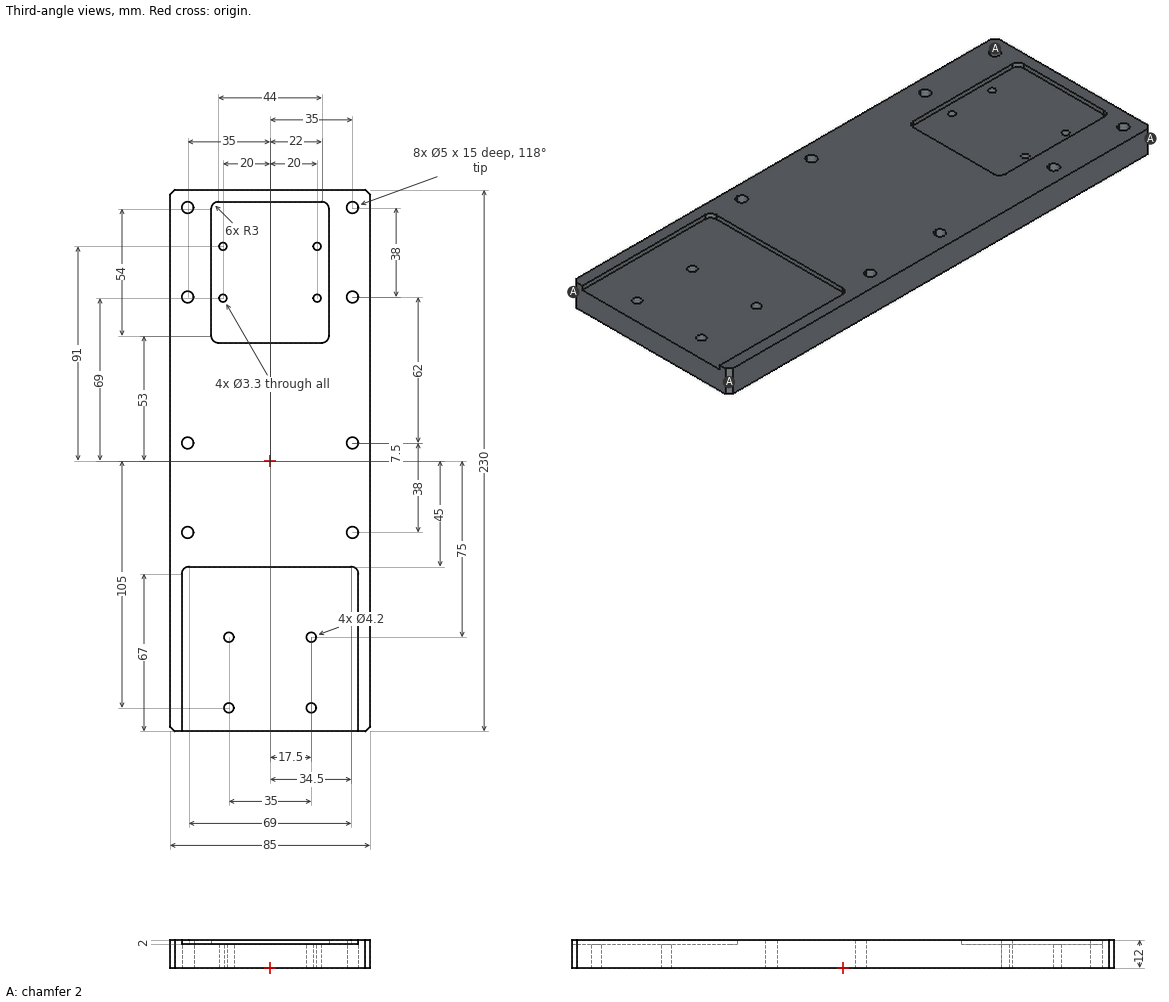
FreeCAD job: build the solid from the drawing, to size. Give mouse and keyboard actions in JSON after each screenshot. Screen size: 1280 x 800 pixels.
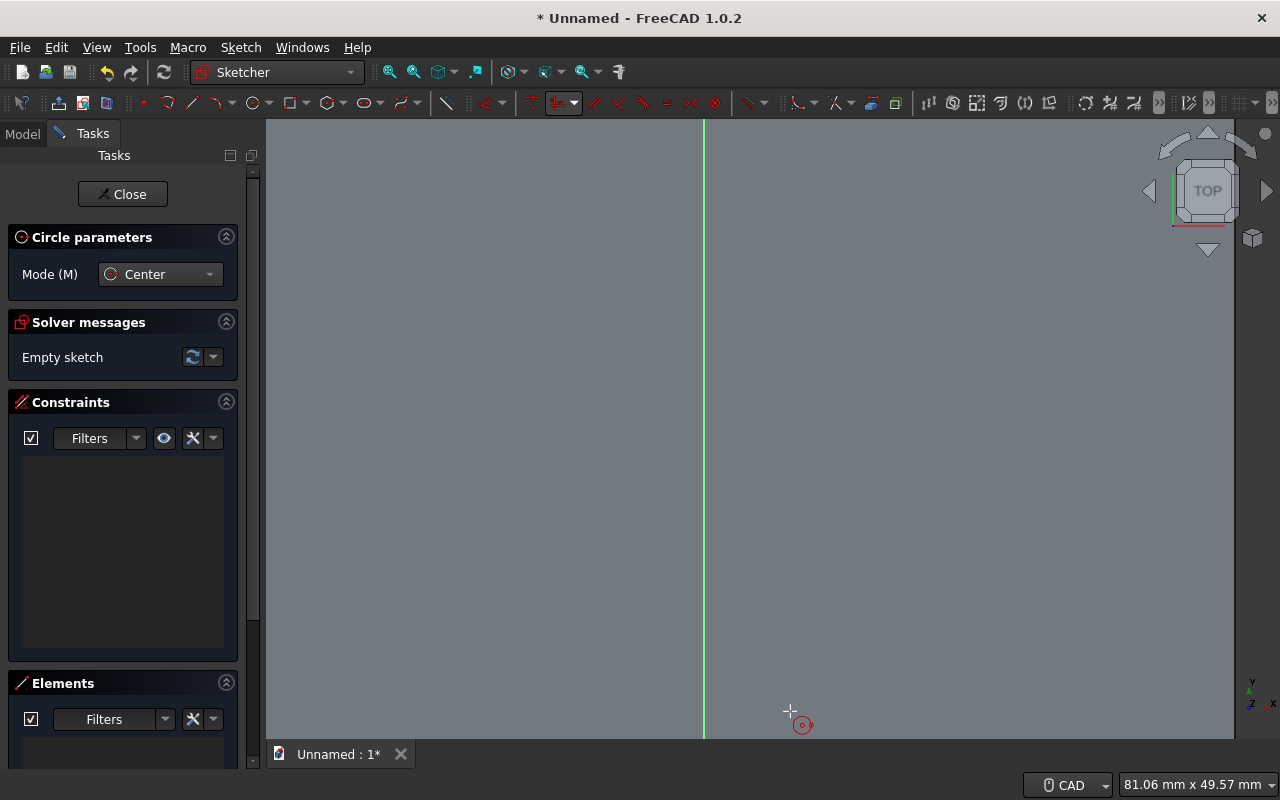
{"action": "left_click", "coordinate": [923, 249]}
{"action": "left_click", "coordinate": [941, 230]}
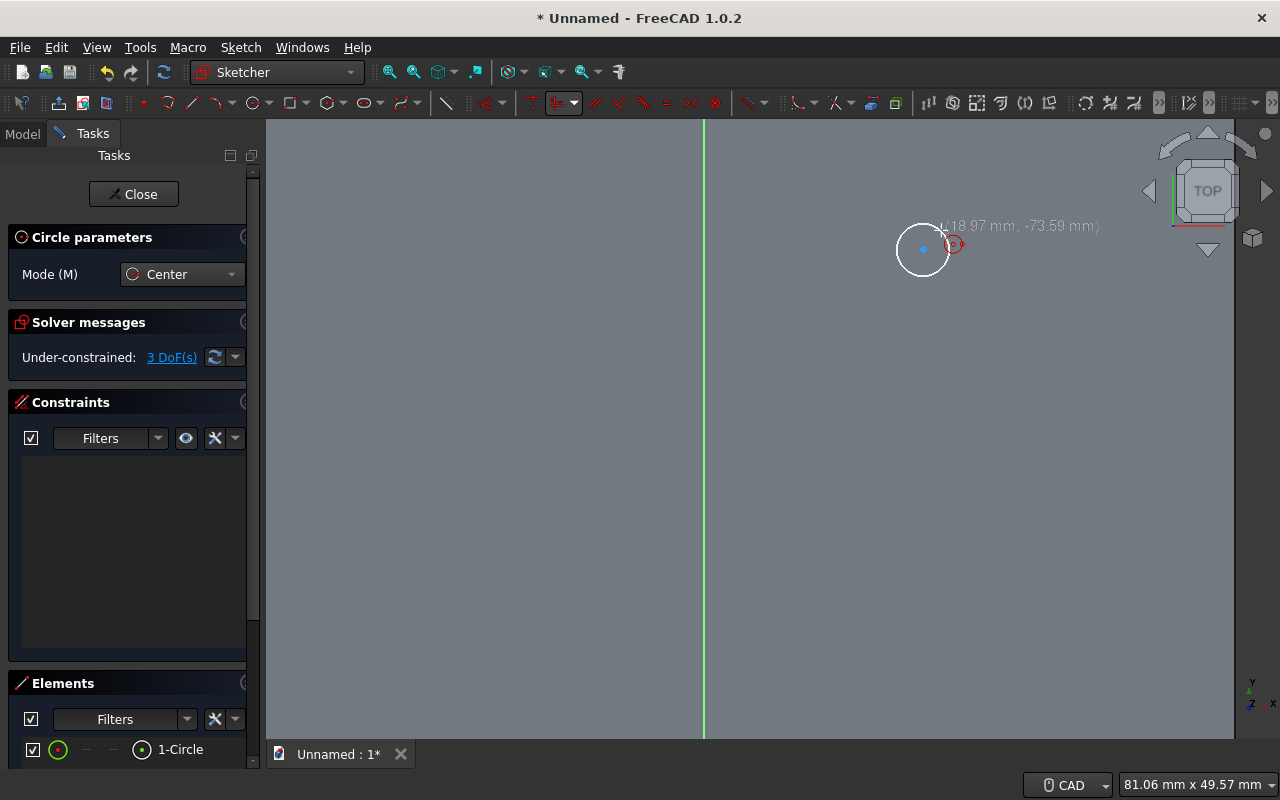
{"action": "left_click", "coordinate": [485, 249]}
{"action": "left_click", "coordinate": [503, 230]}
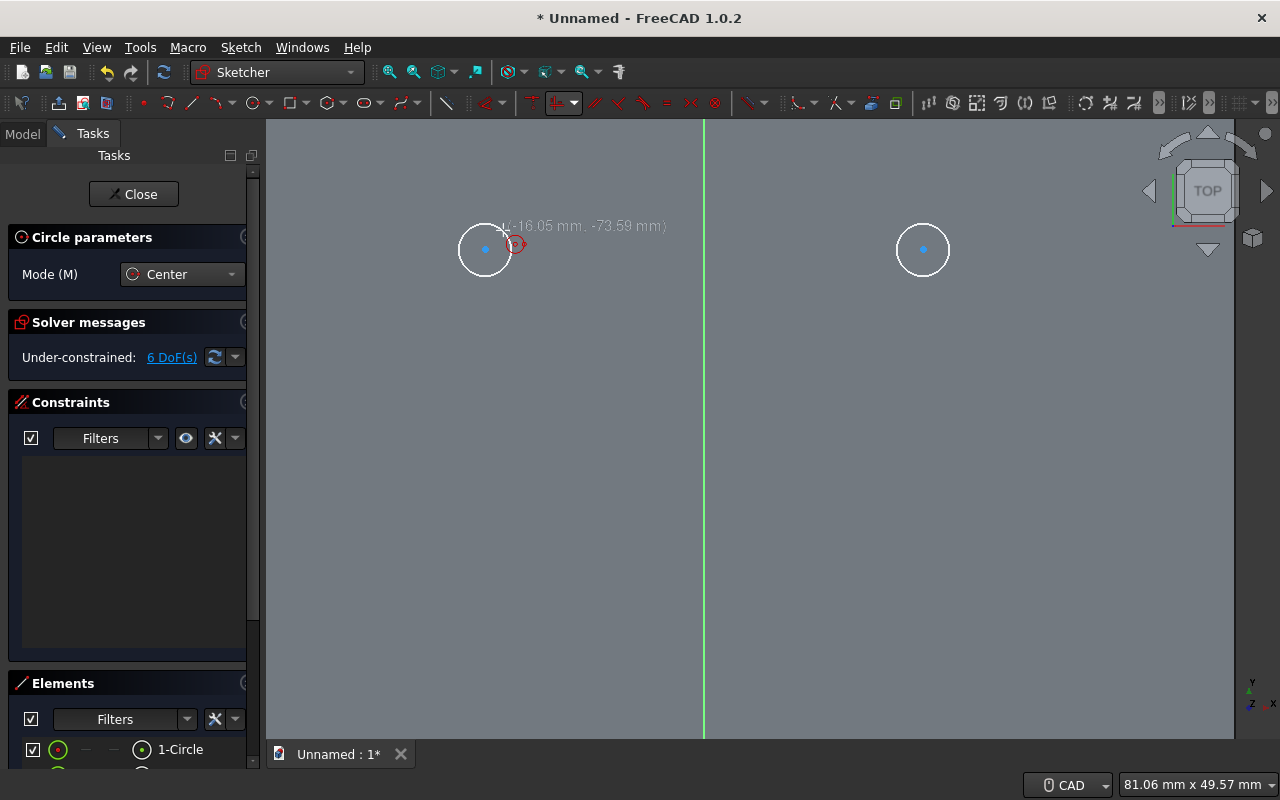
{"action": "left_click", "coordinate": [485, 624]}
{"action": "left_click", "coordinate": [503, 605]}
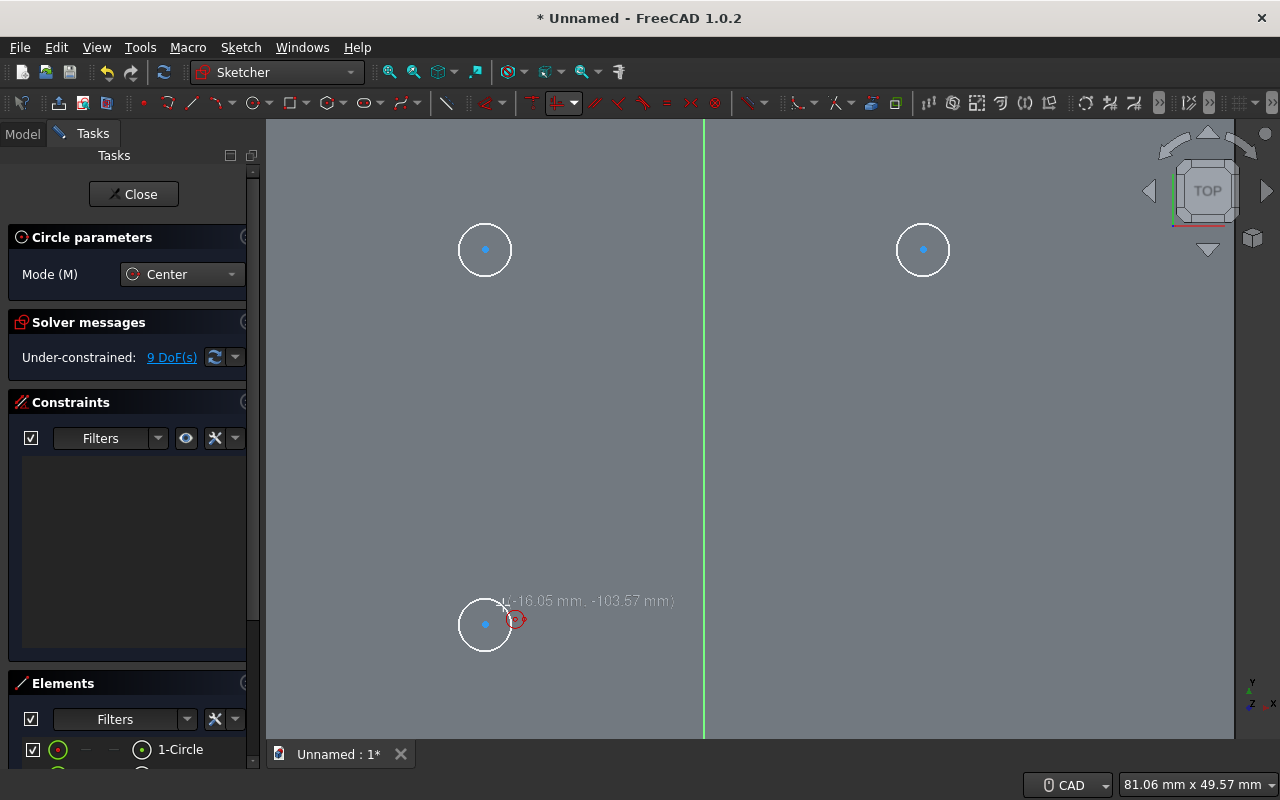
{"action": "left_click", "coordinate": [923, 624]}
{"action": "left_click", "coordinate": [941, 605]}
{"action": "key", "text": "Escape"}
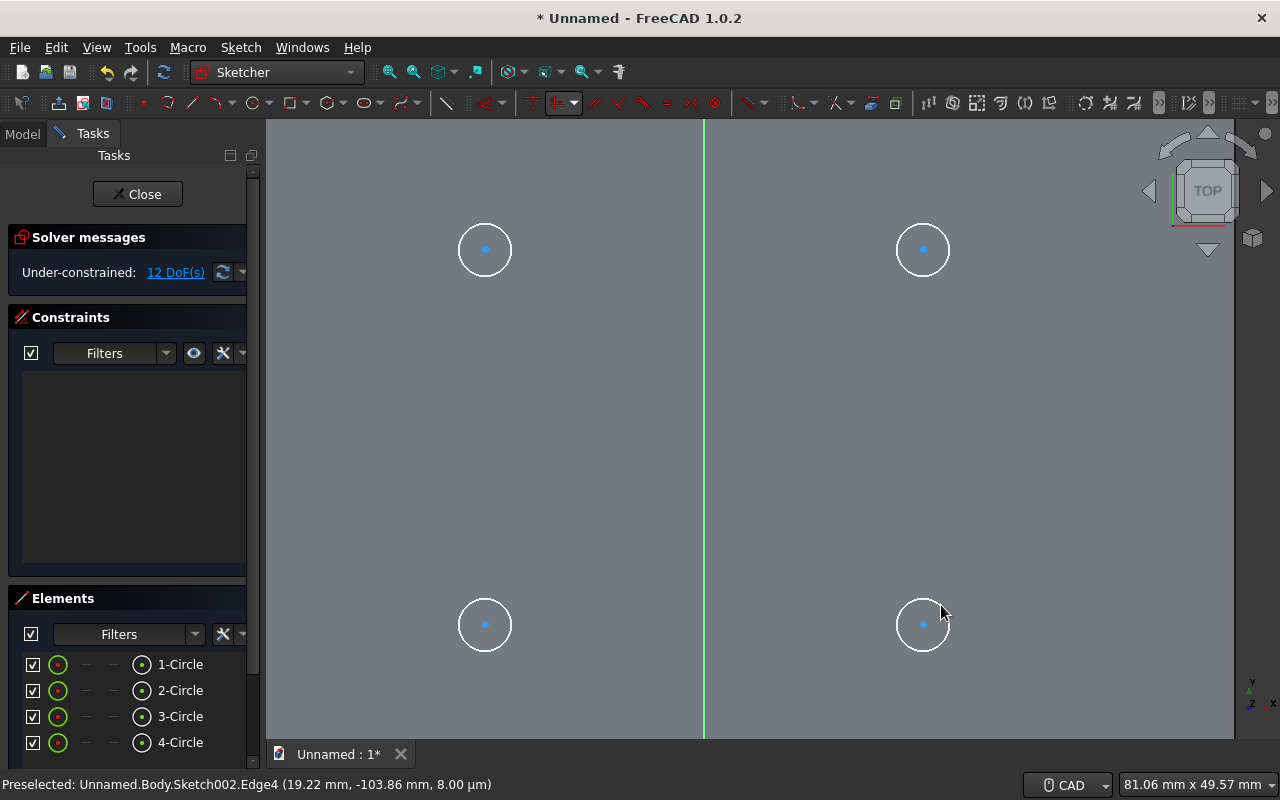
{"action": "left_click", "coordinate": [941, 231]}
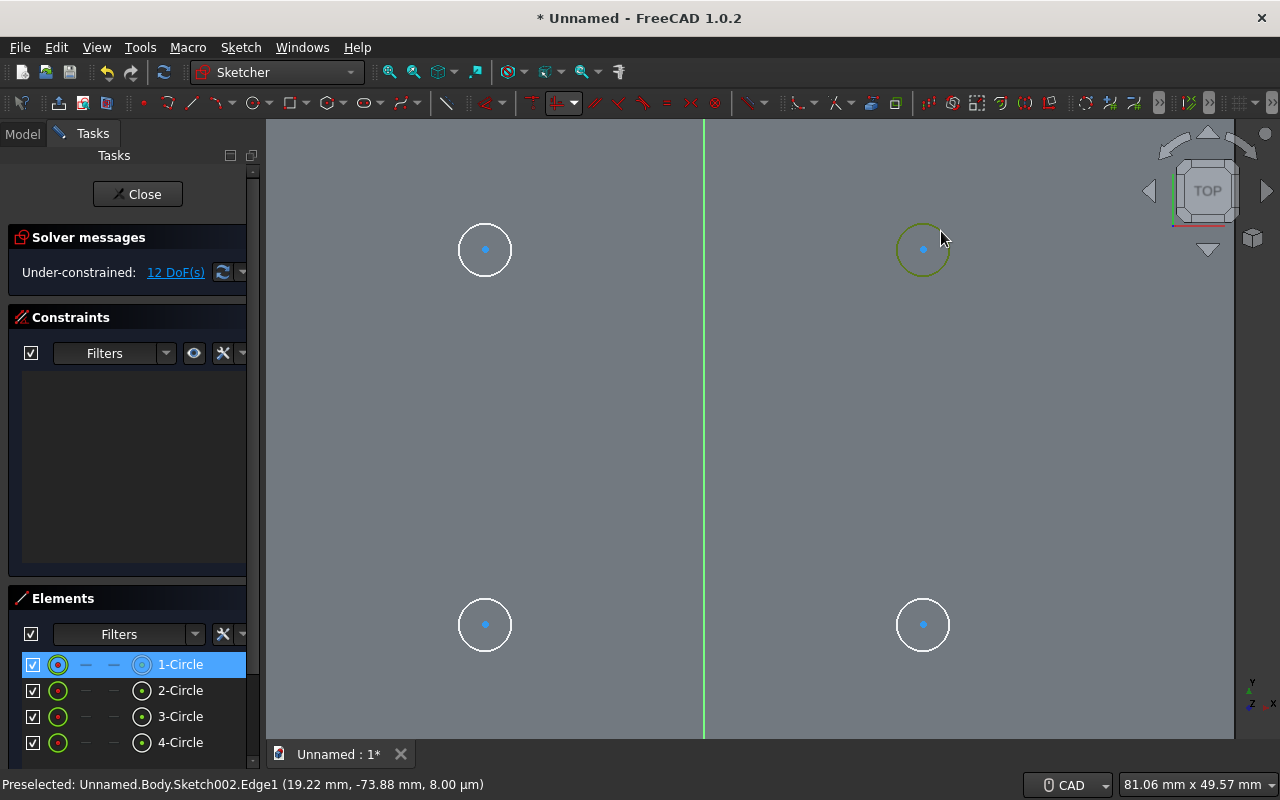
{"action": "left_click", "coordinate": [503, 231]}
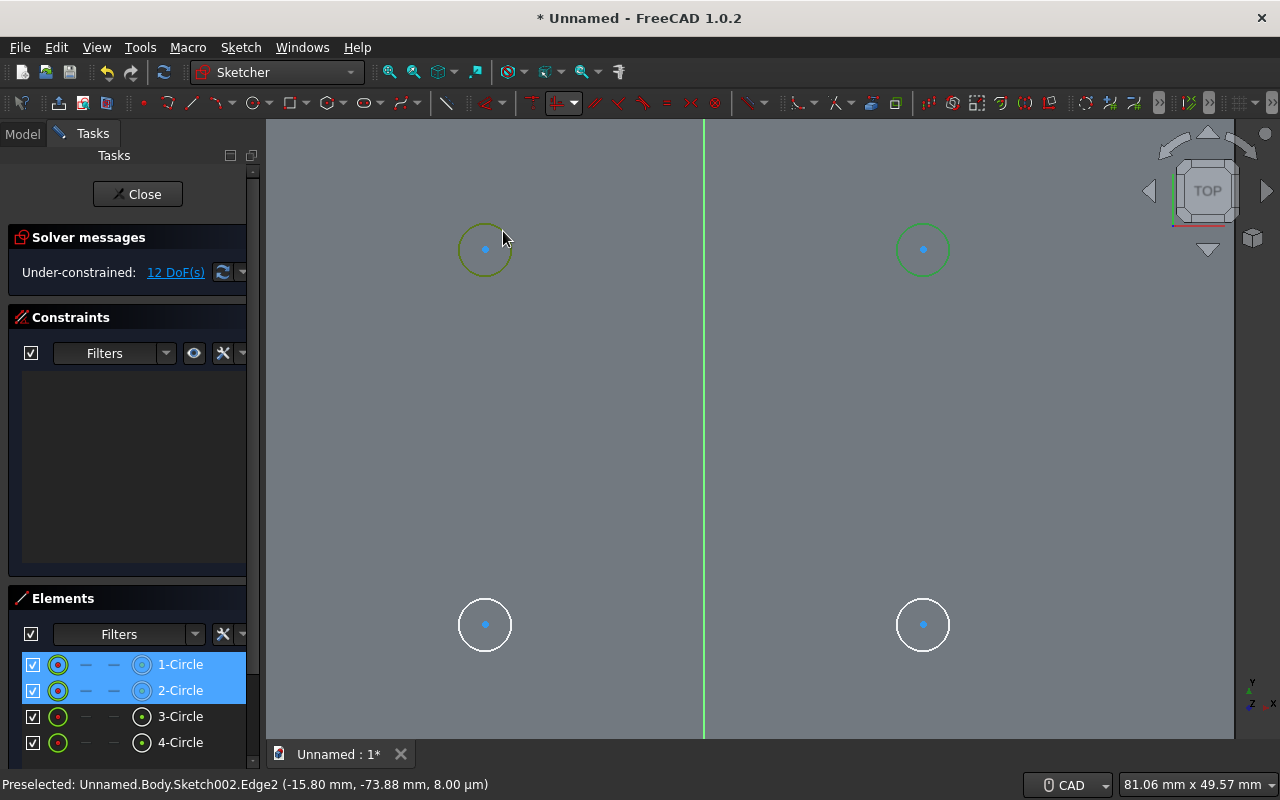
{"action": "left_click", "coordinate": [503, 606]}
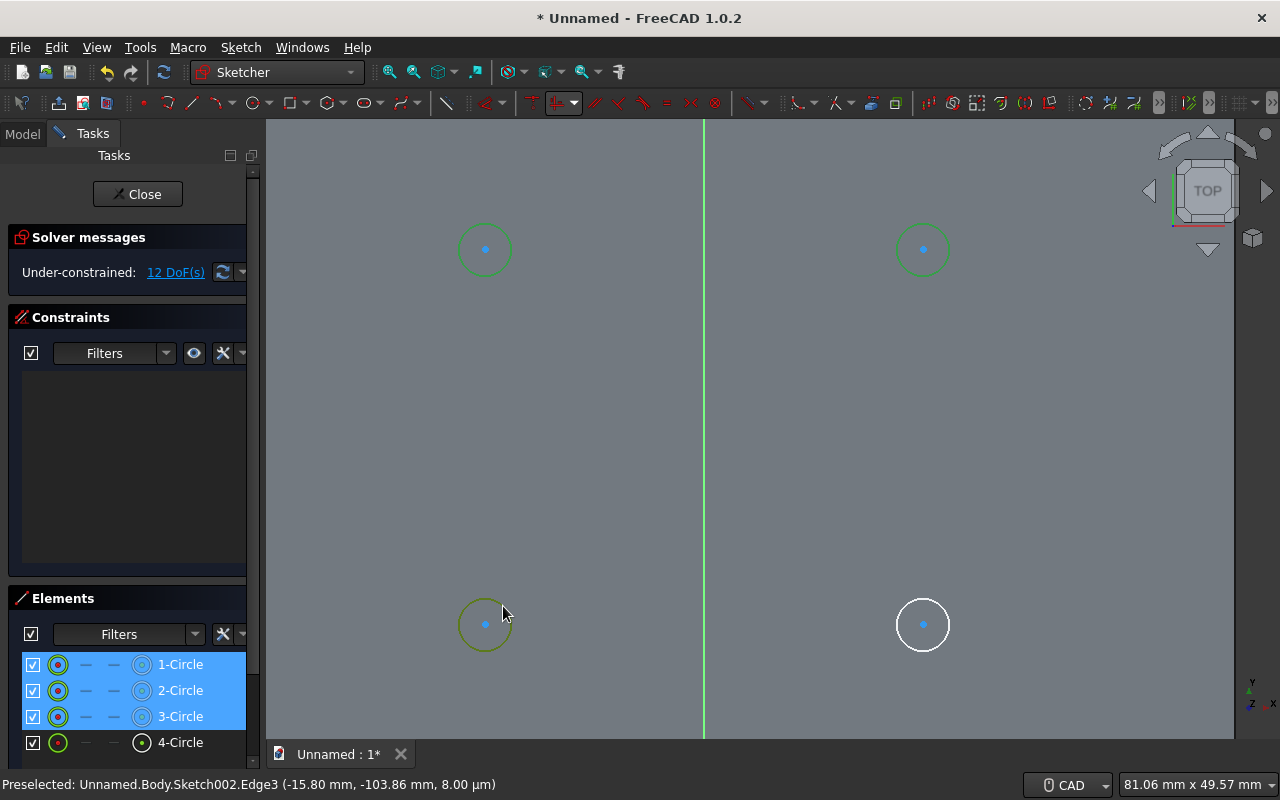
{"action": "left_click", "coordinate": [941, 606]}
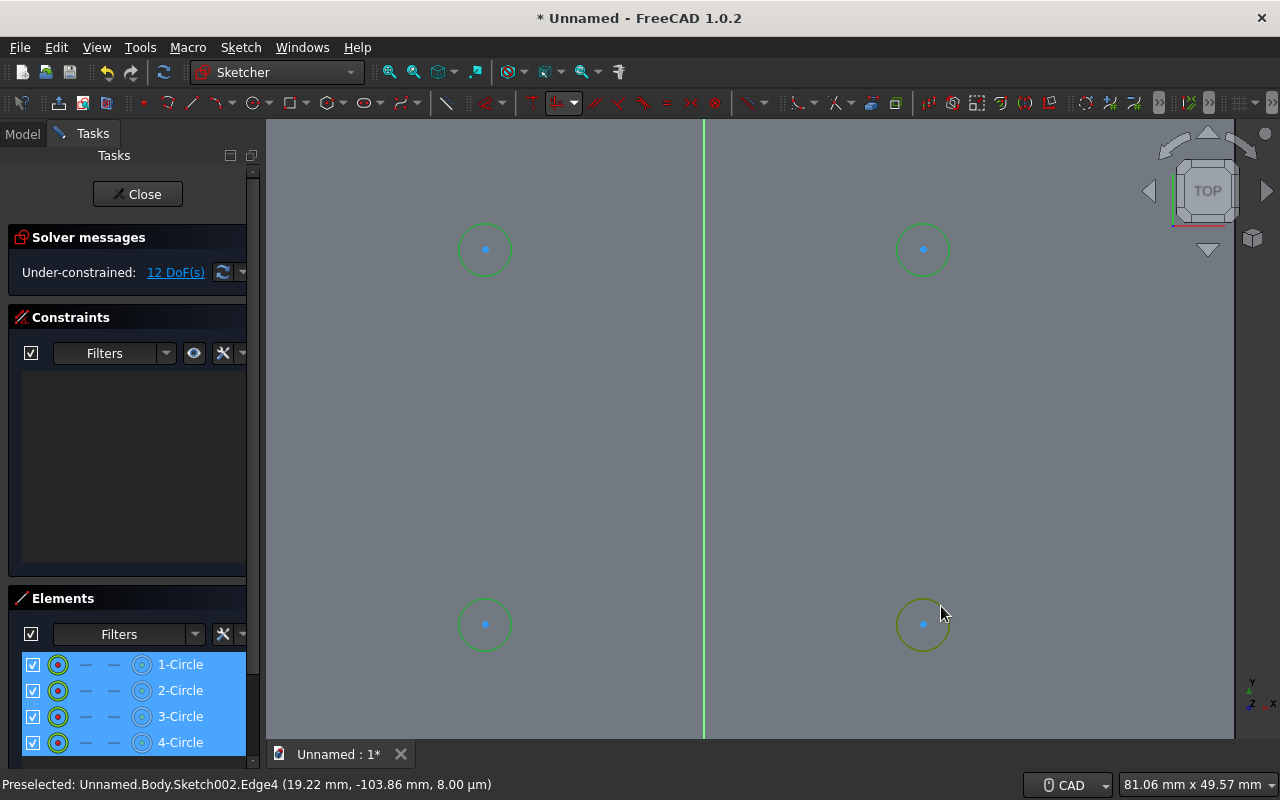
{"action": "key", "text": "e"}